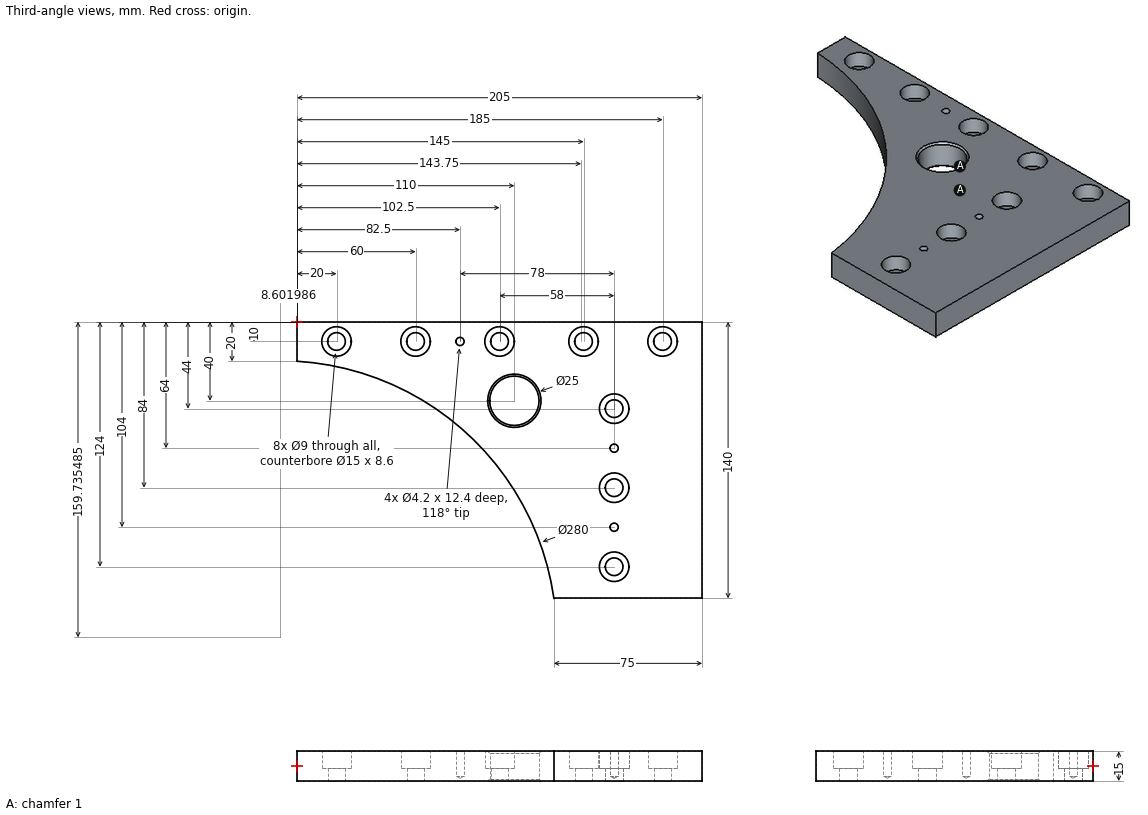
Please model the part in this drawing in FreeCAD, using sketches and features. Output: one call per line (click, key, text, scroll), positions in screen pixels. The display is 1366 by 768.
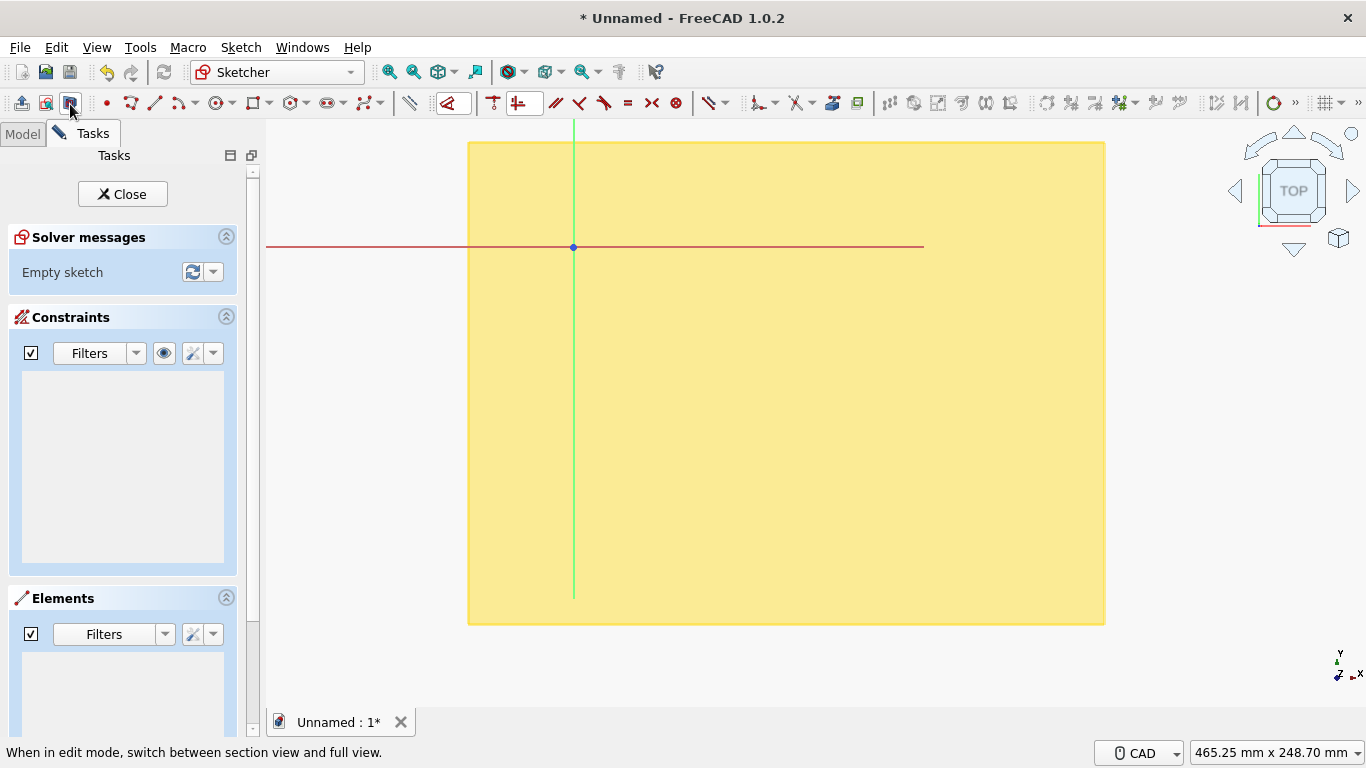
scroll(851, 328, up, 9)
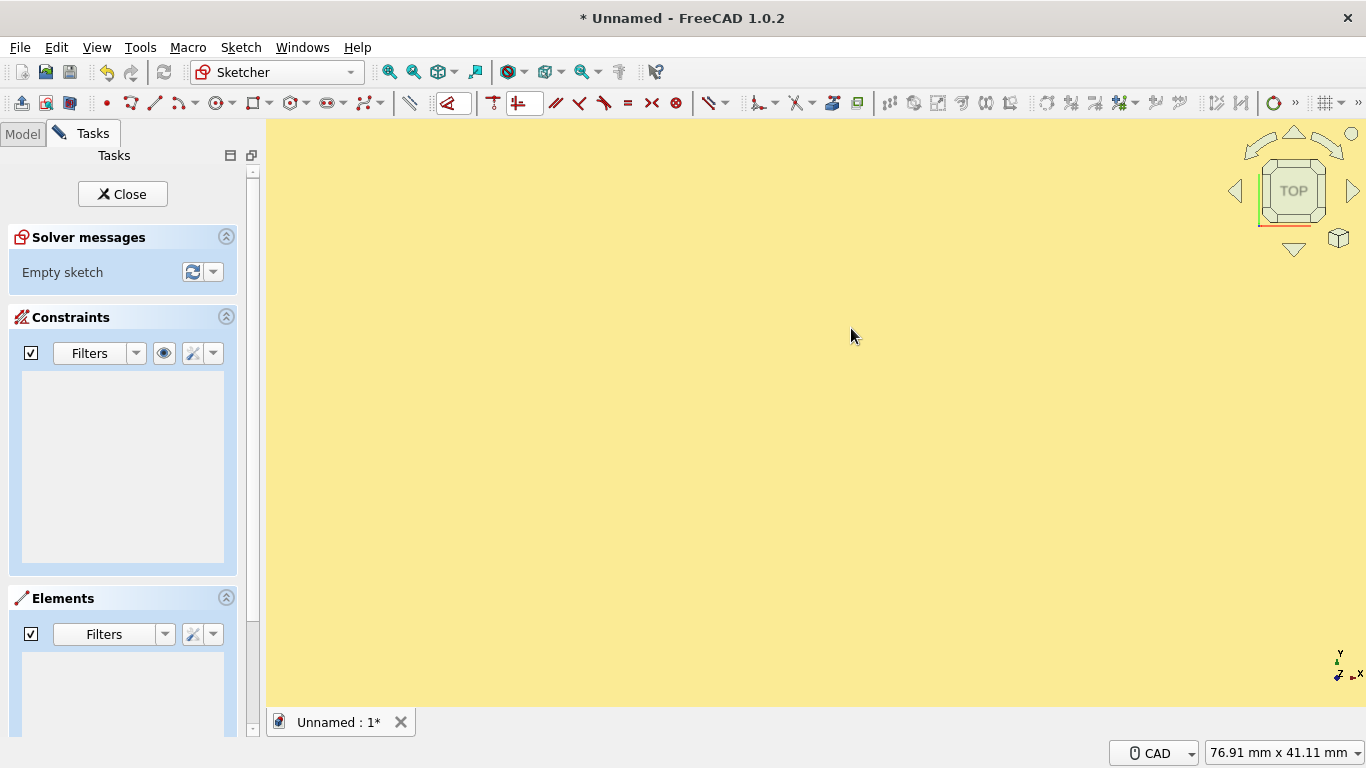
click(216, 104)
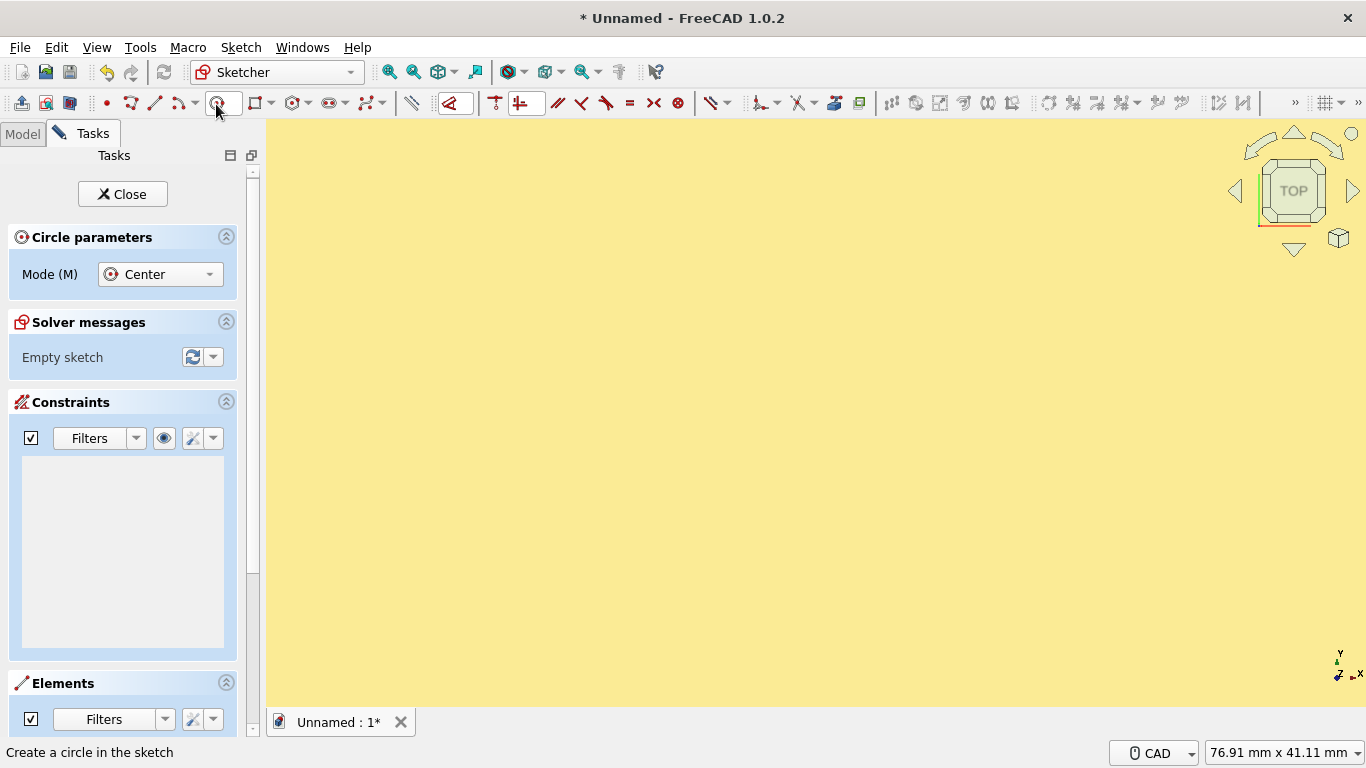
click(744, 411)
click(870, 285)
key(Escape)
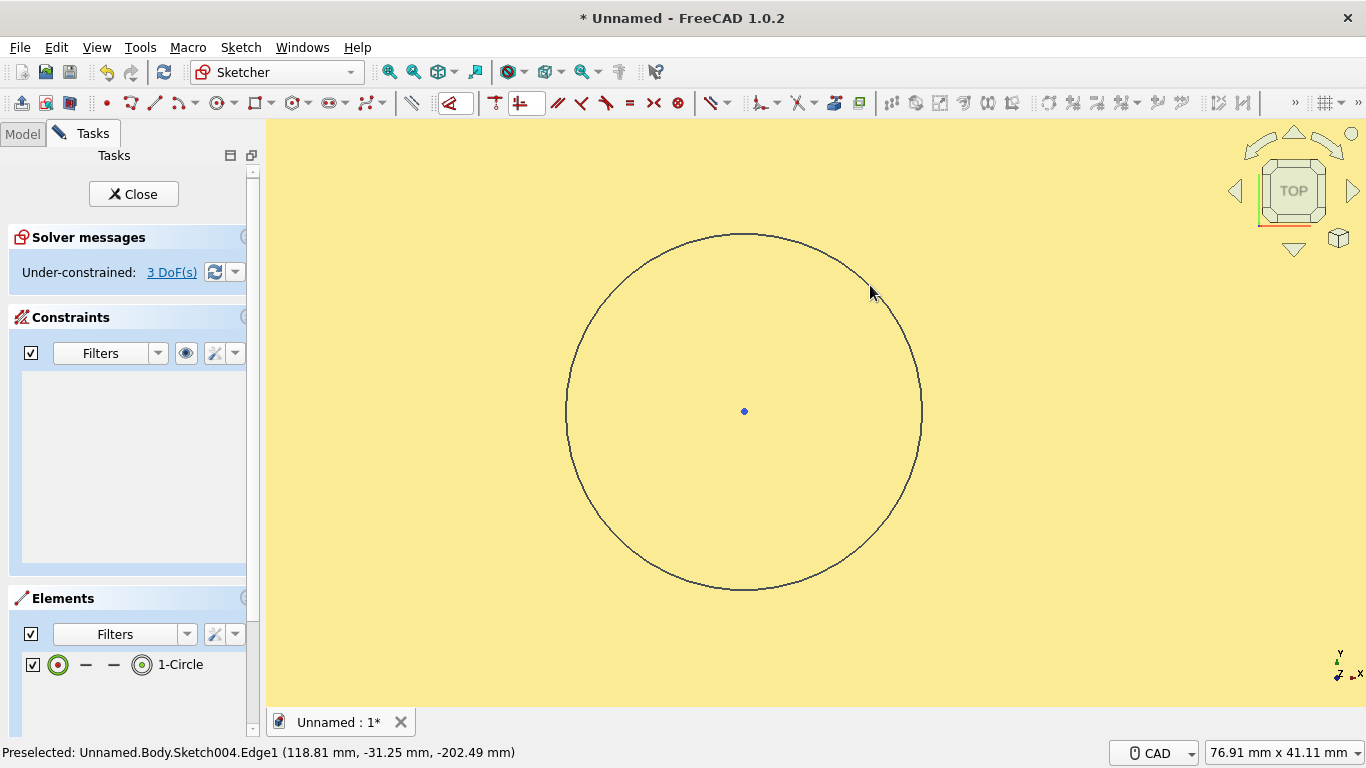
click(870, 286)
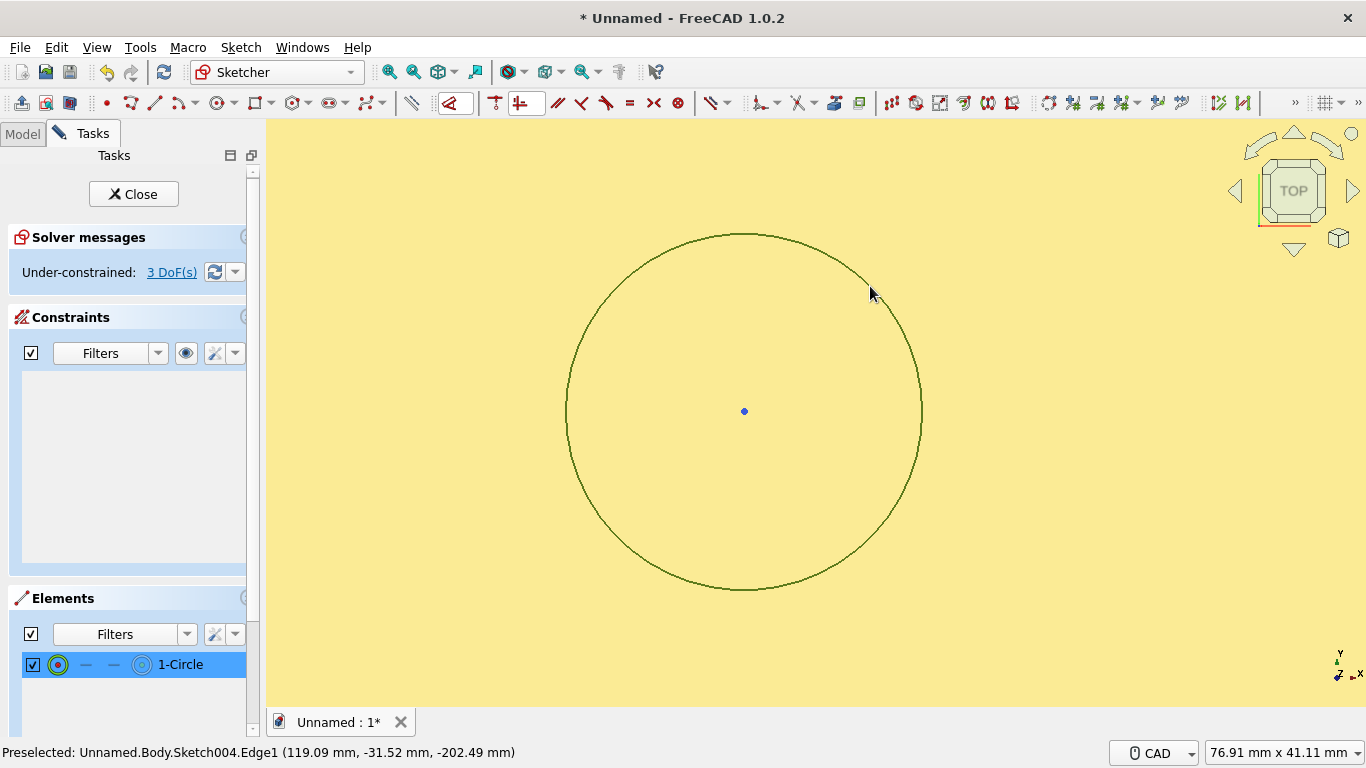
click(468, 104)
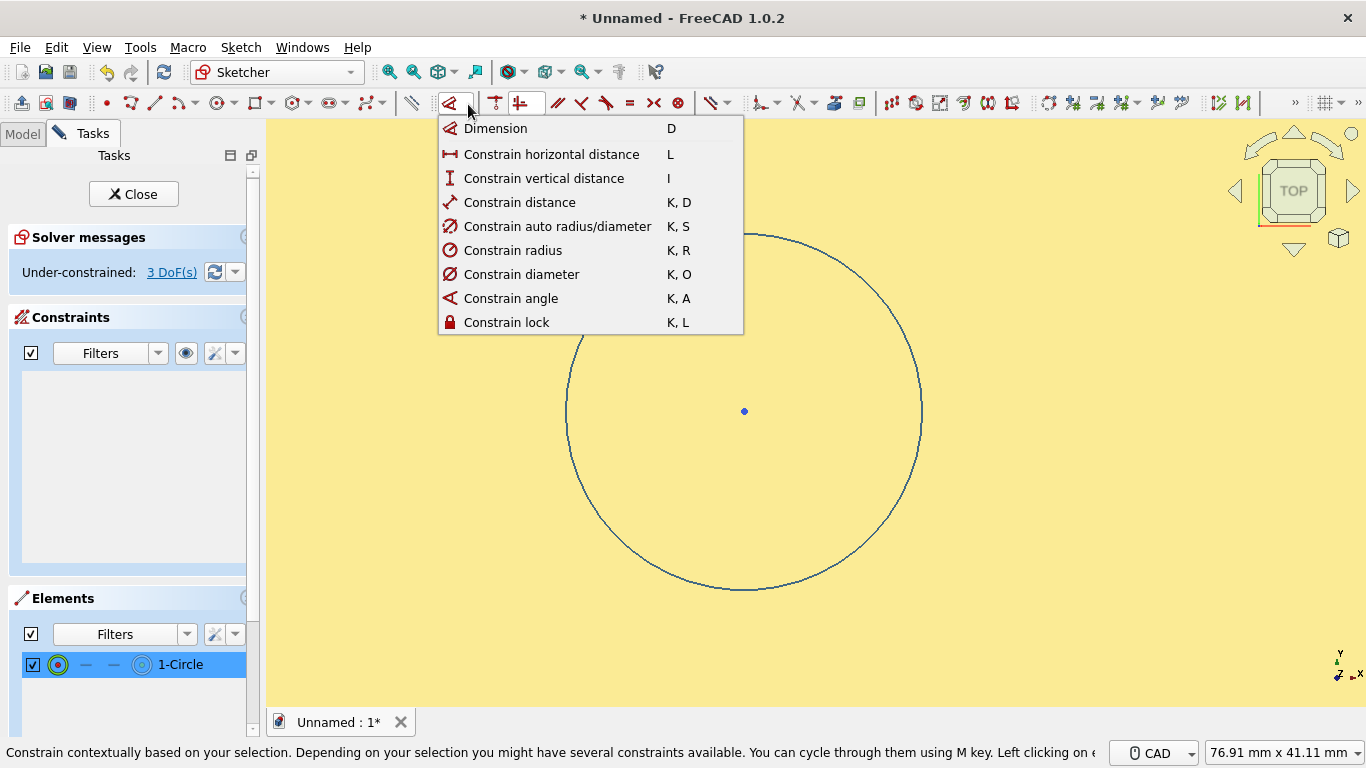
click(591, 274)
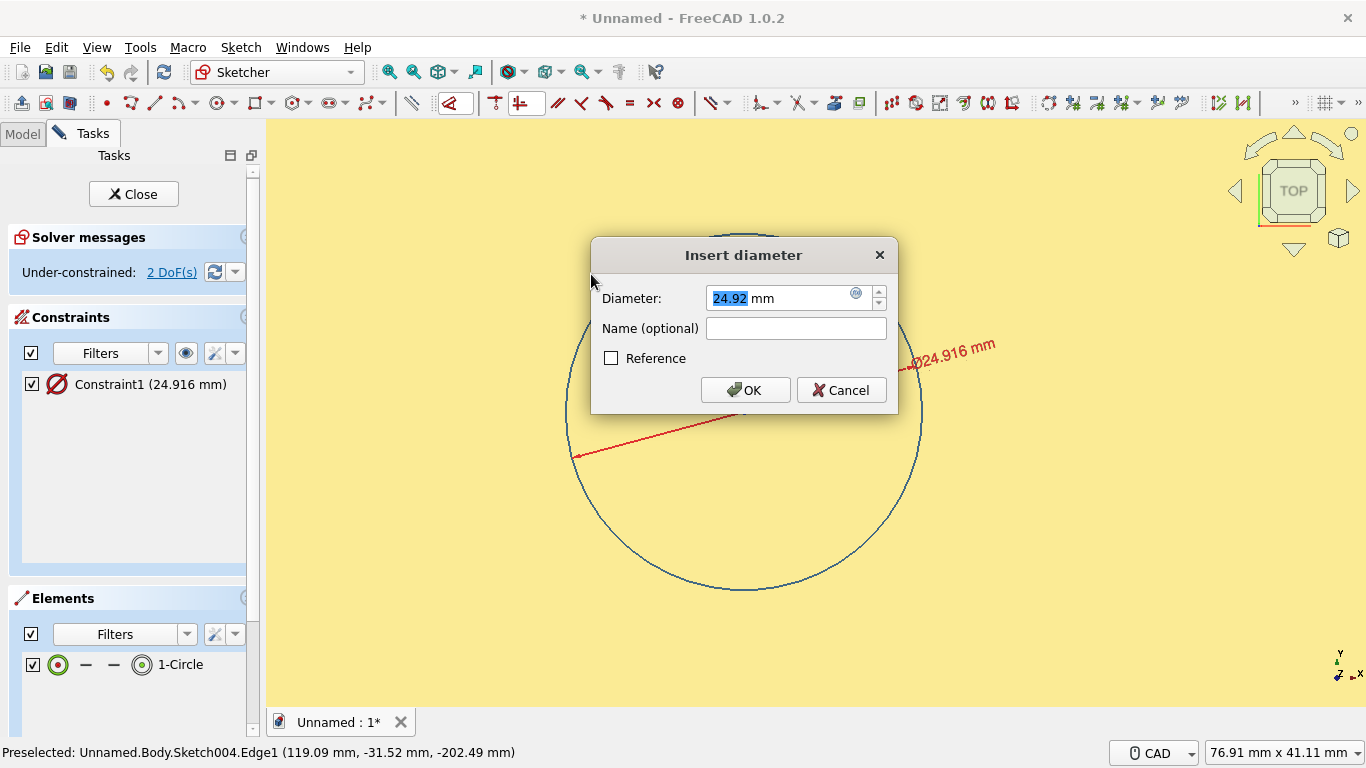
text(25)
key(Return)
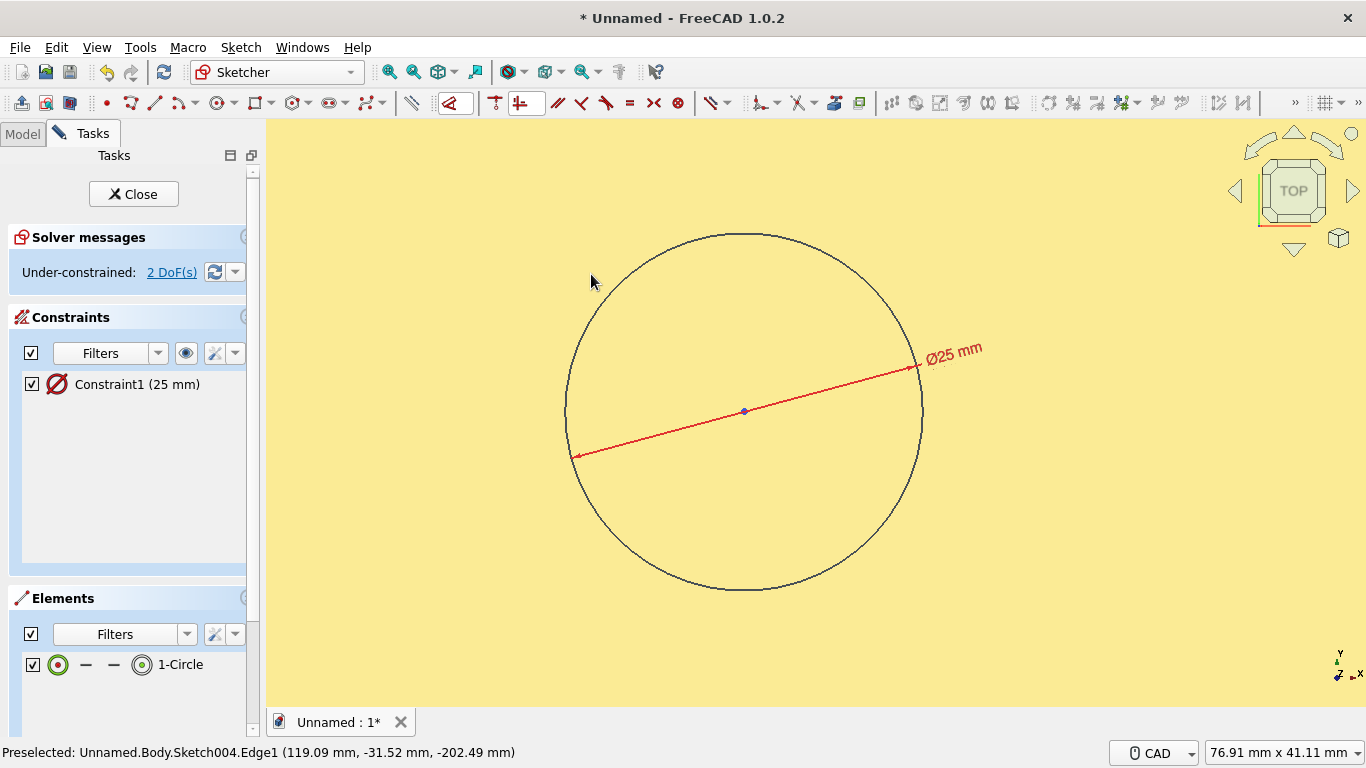
click(744, 412)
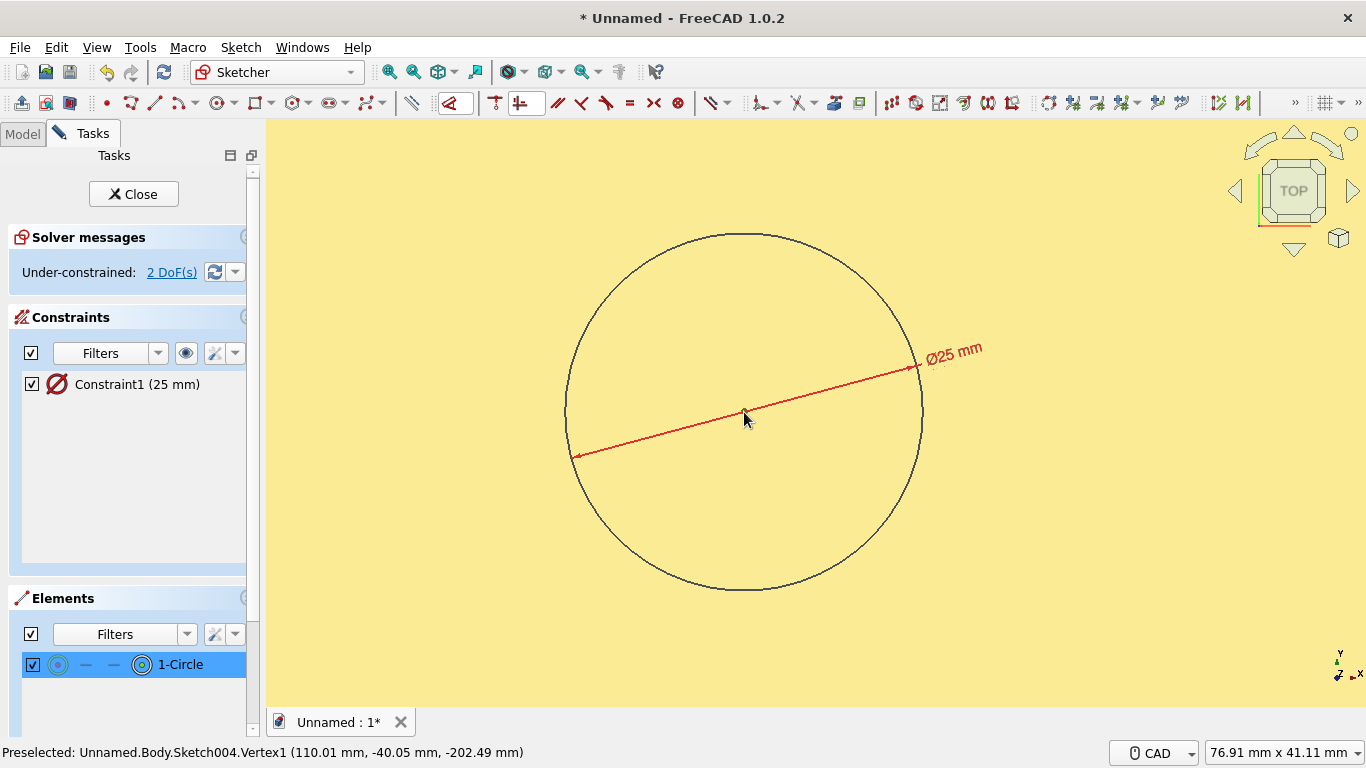
click(468, 104)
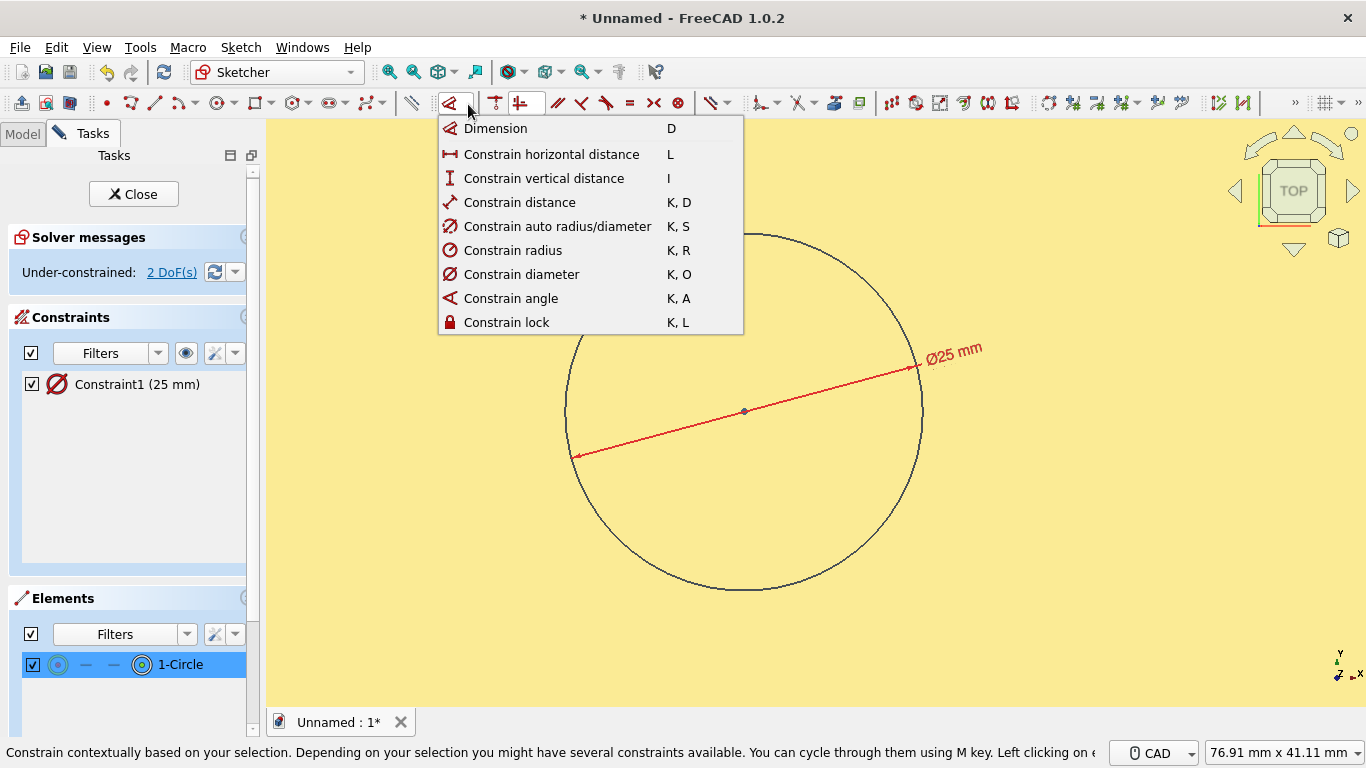
click(591, 178)